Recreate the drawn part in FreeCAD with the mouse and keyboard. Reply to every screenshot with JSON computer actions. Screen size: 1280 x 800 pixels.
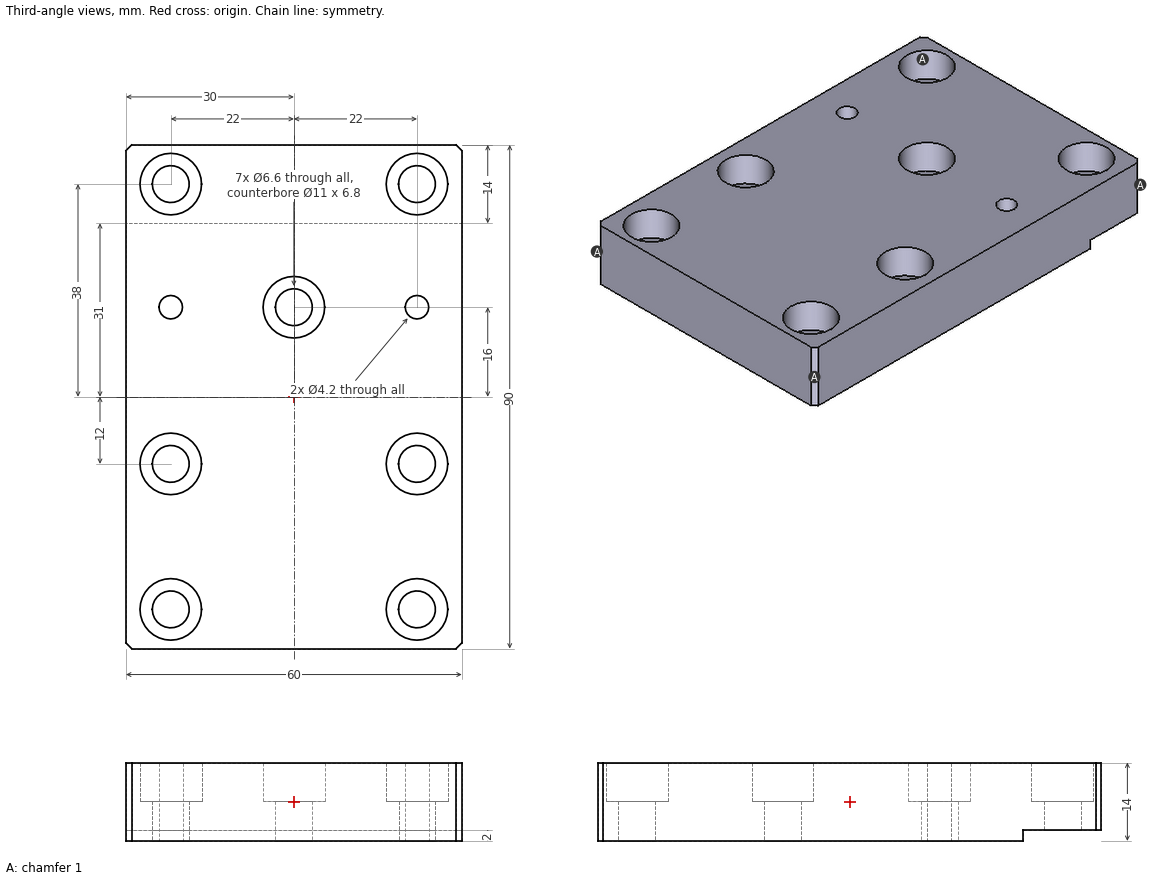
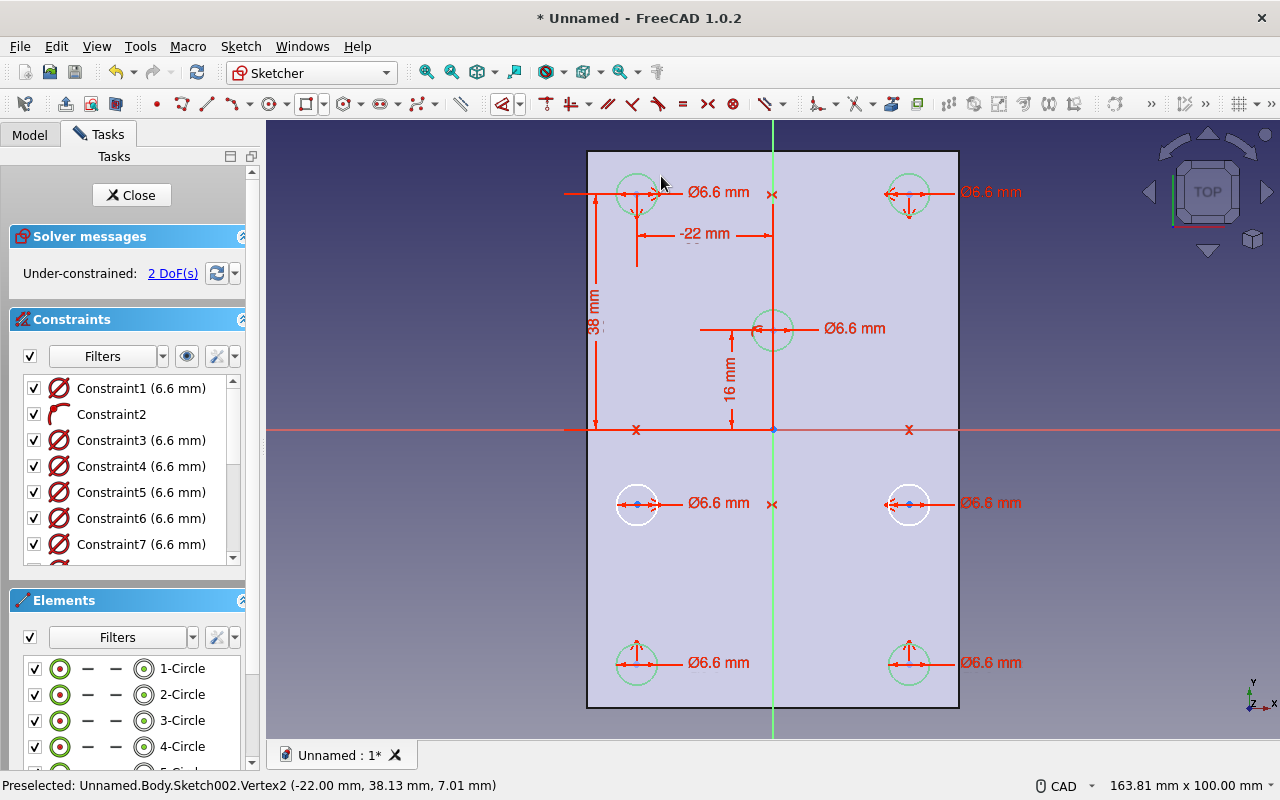
{"action": "left_click", "coordinate": [637, 505]}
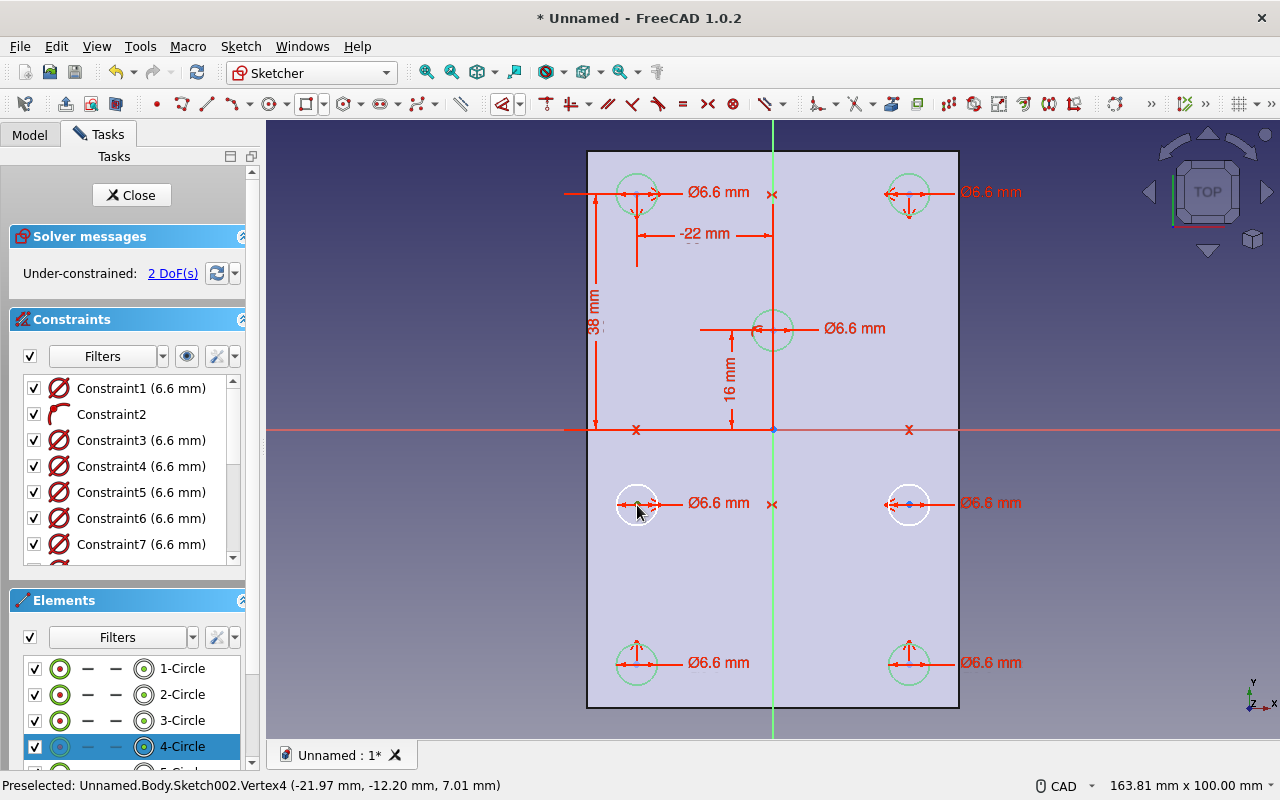
{"action": "left_click", "coordinate": [520, 104]}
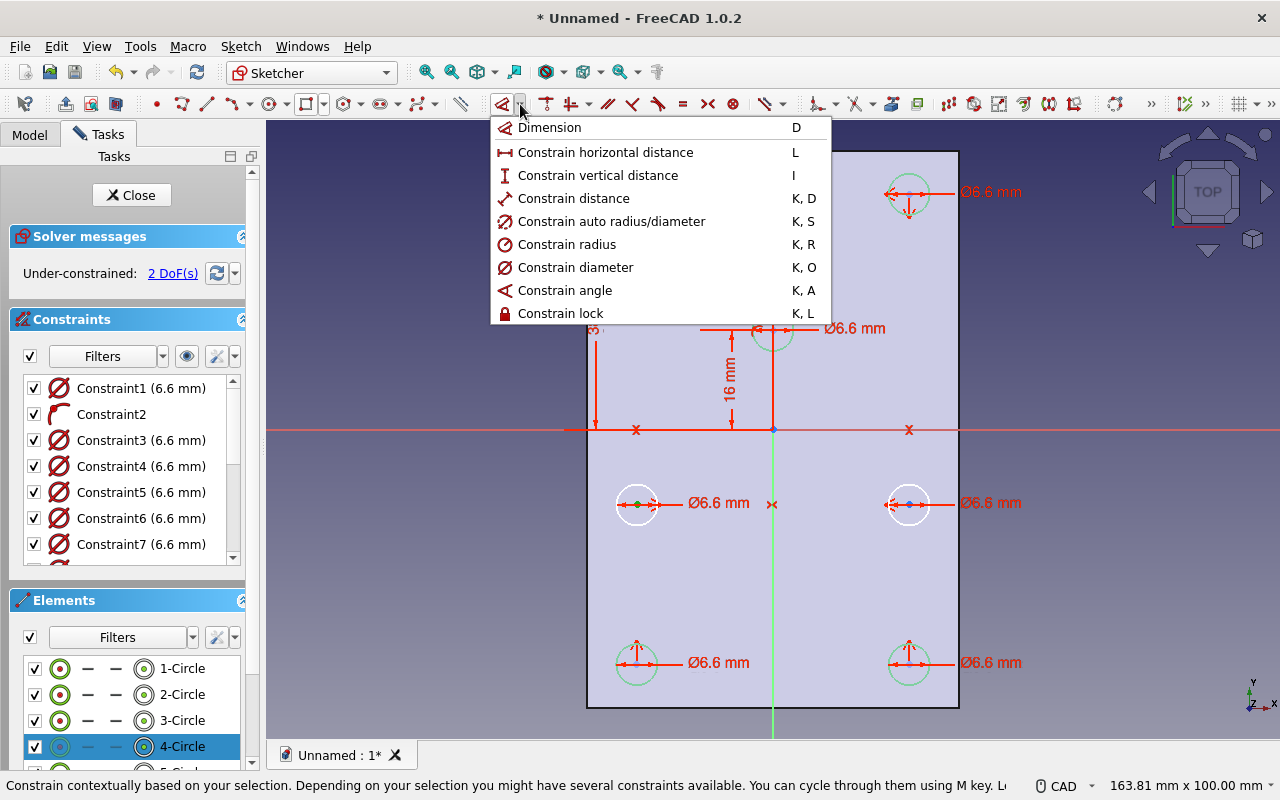
{"action": "left_click", "coordinate": [661, 152]}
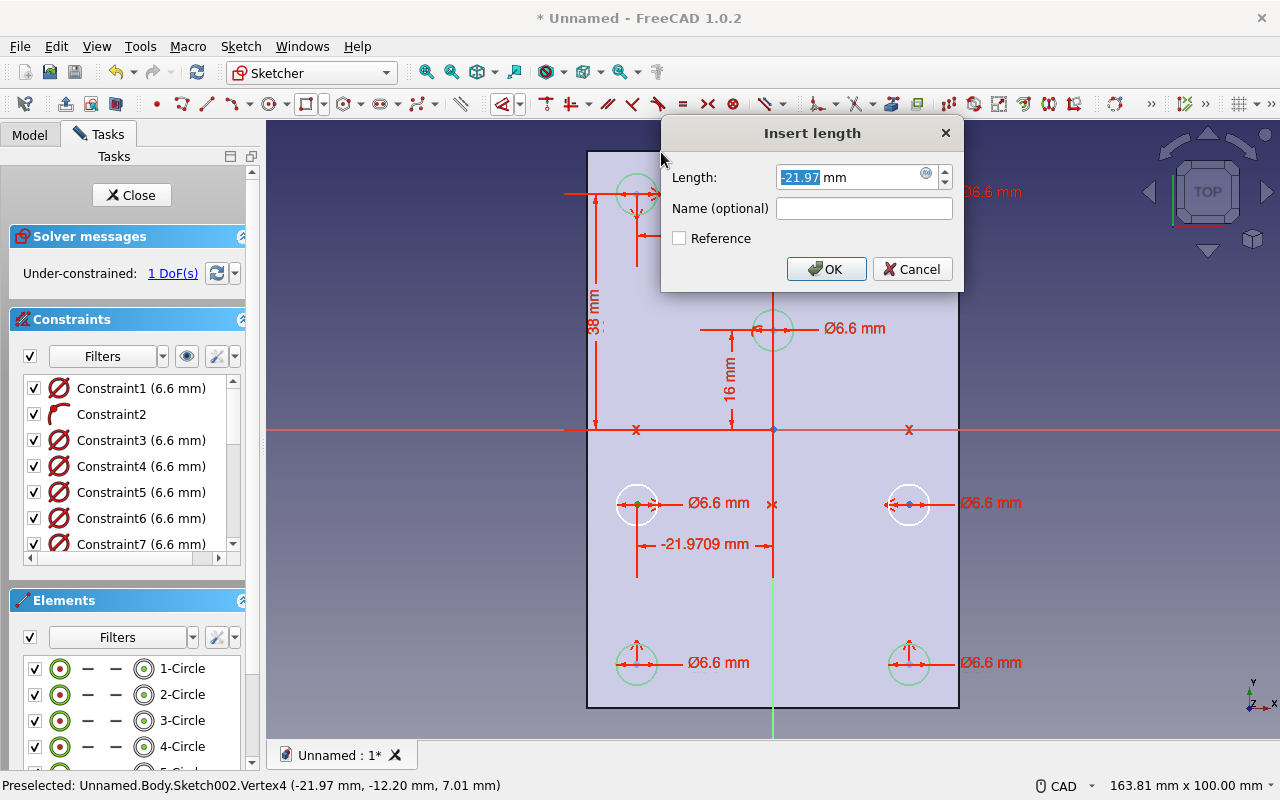
{"action": "type", "text": "-22"}
{"action": "key", "text": "Return"}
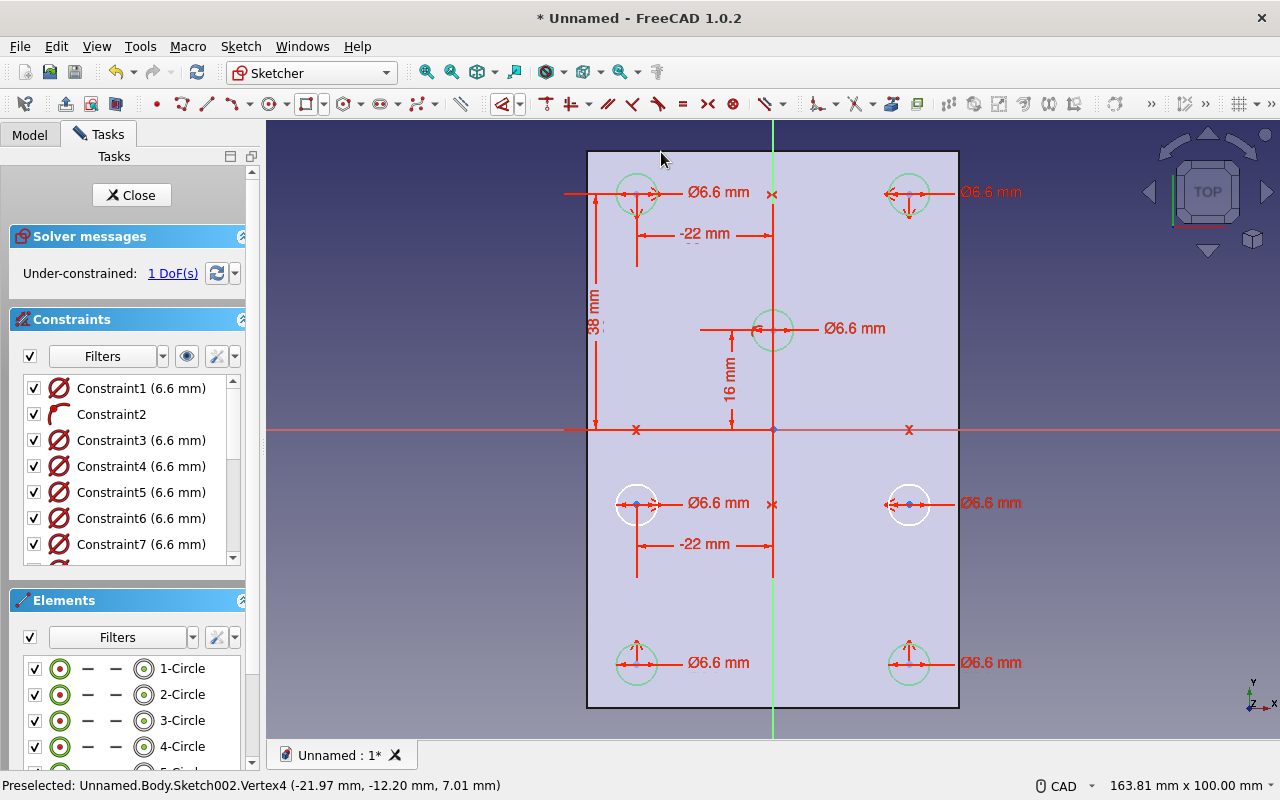
{"action": "left_click", "coordinate": [637, 505]}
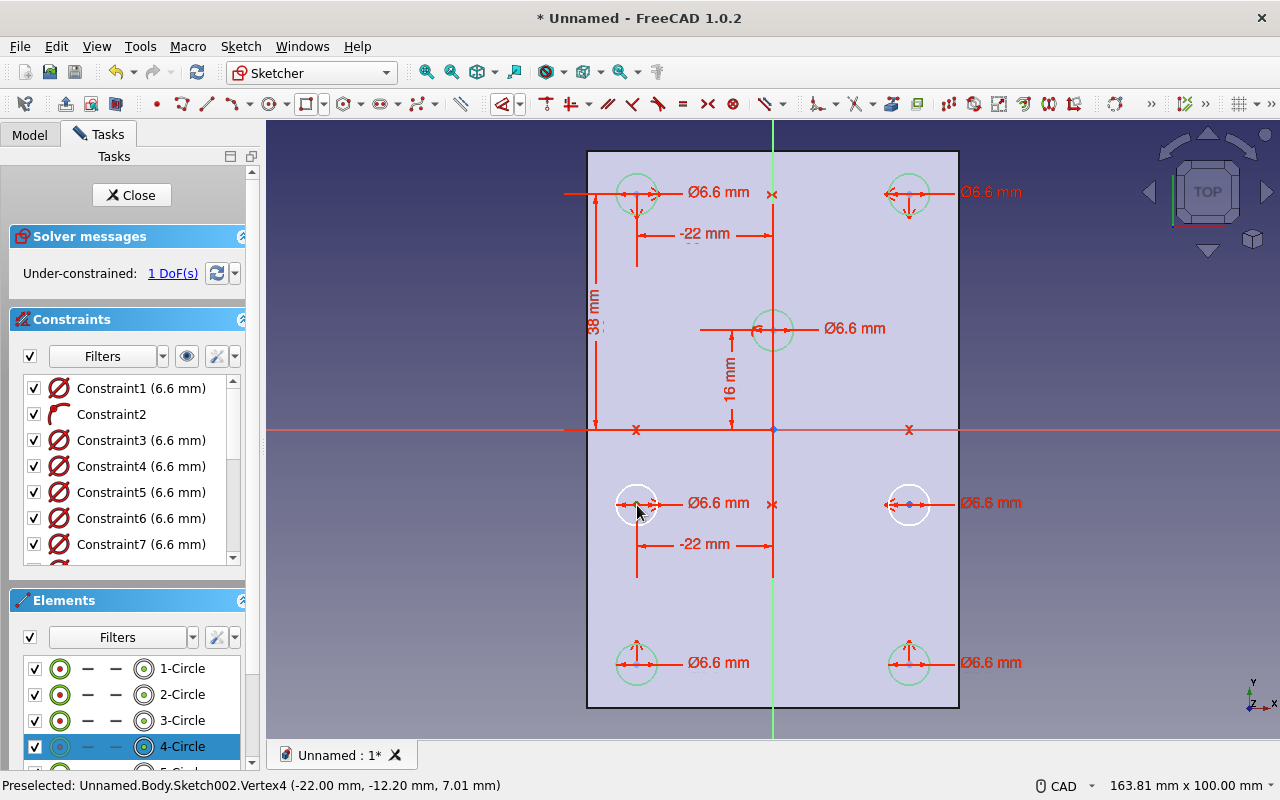
{"action": "left_click", "coordinate": [520, 104]}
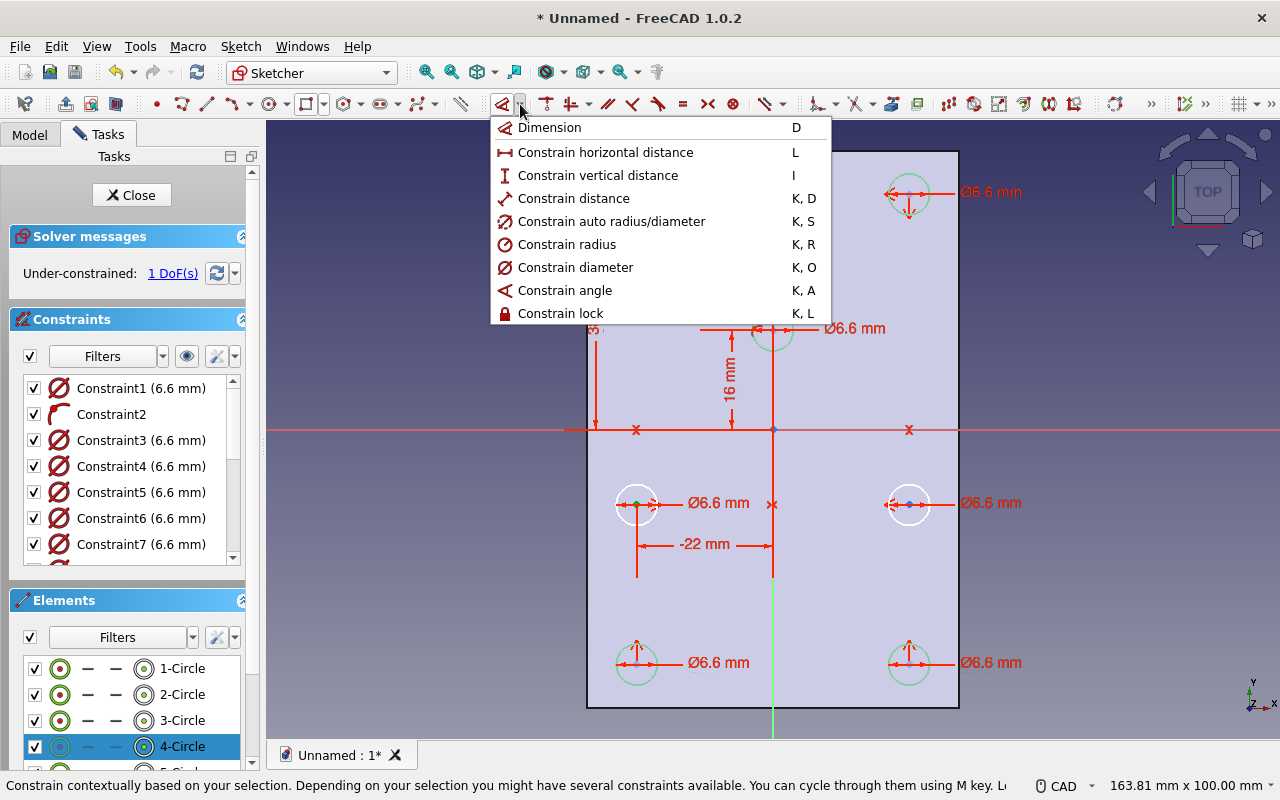
{"action": "left_click", "coordinate": [661, 176]}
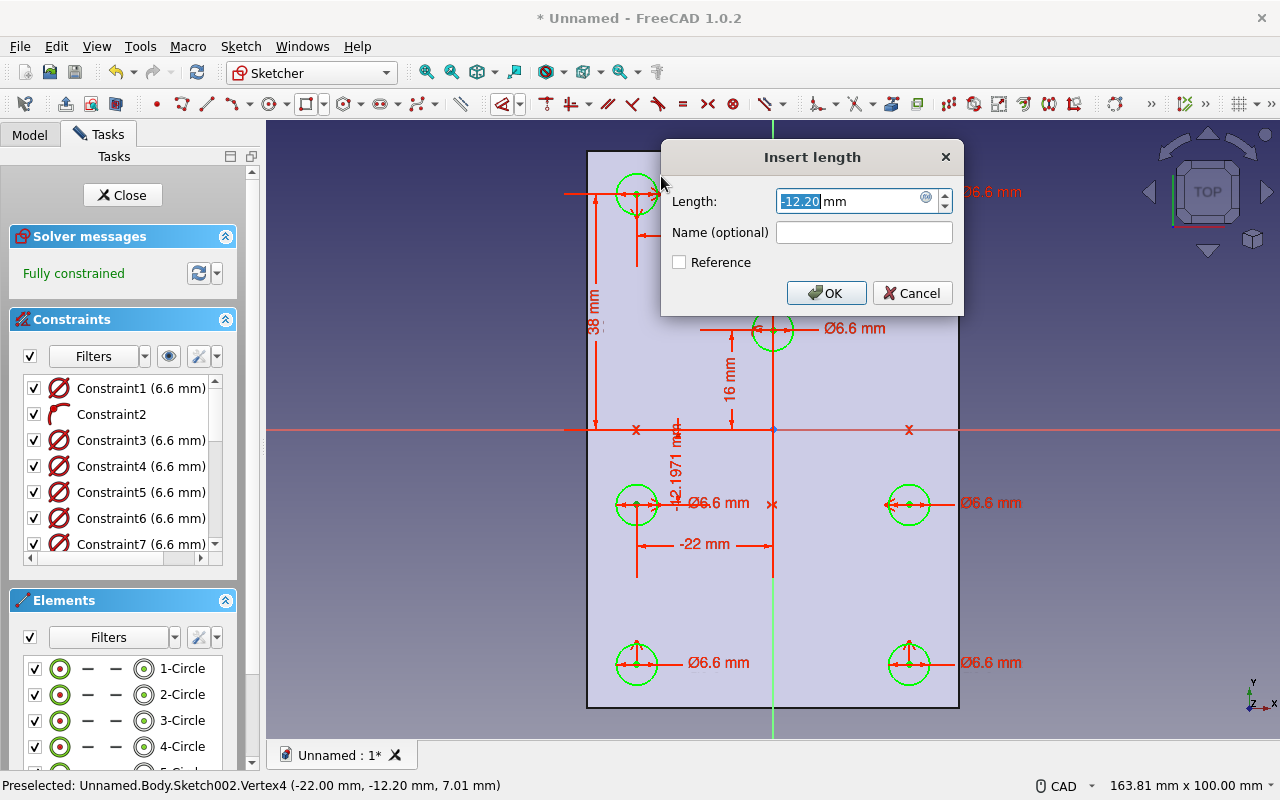
{"action": "type", "text": "-12"}
{"action": "key", "text": "Return"}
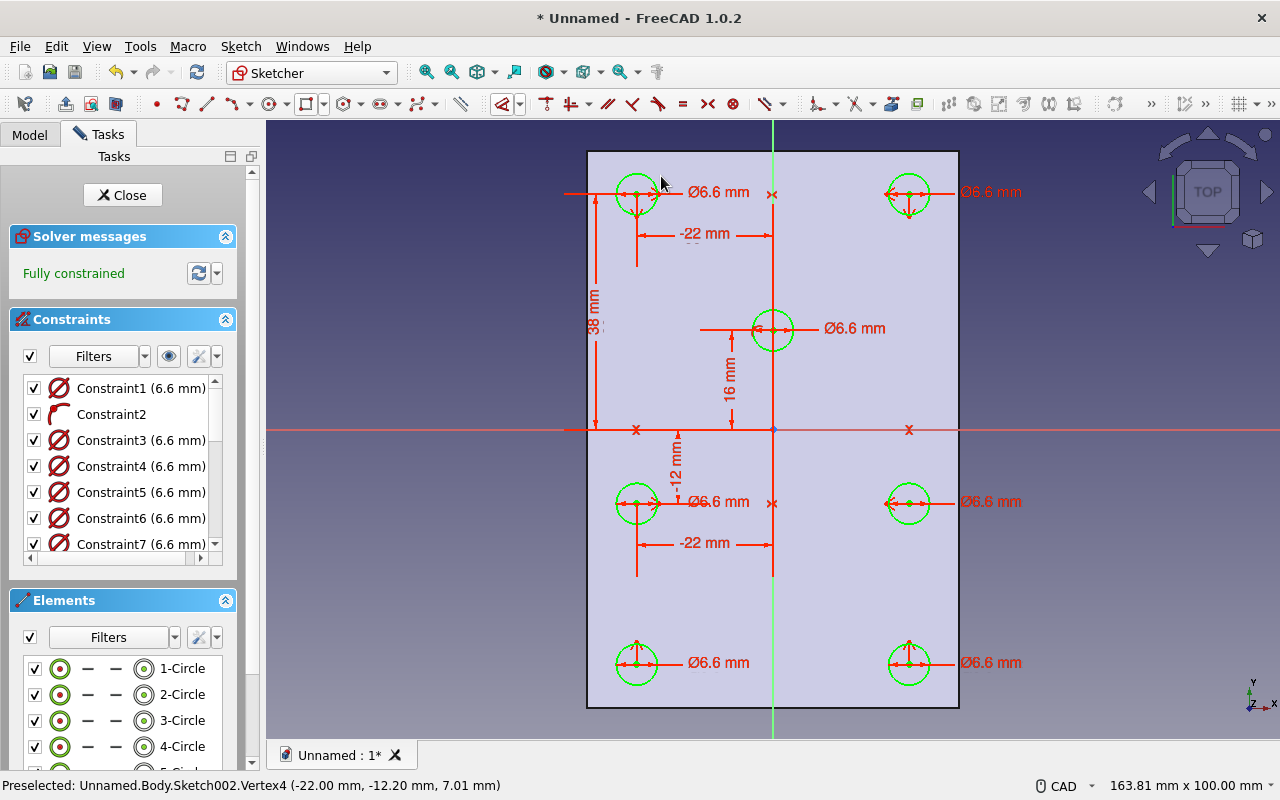
{"action": "left_click", "coordinate": [123, 195]}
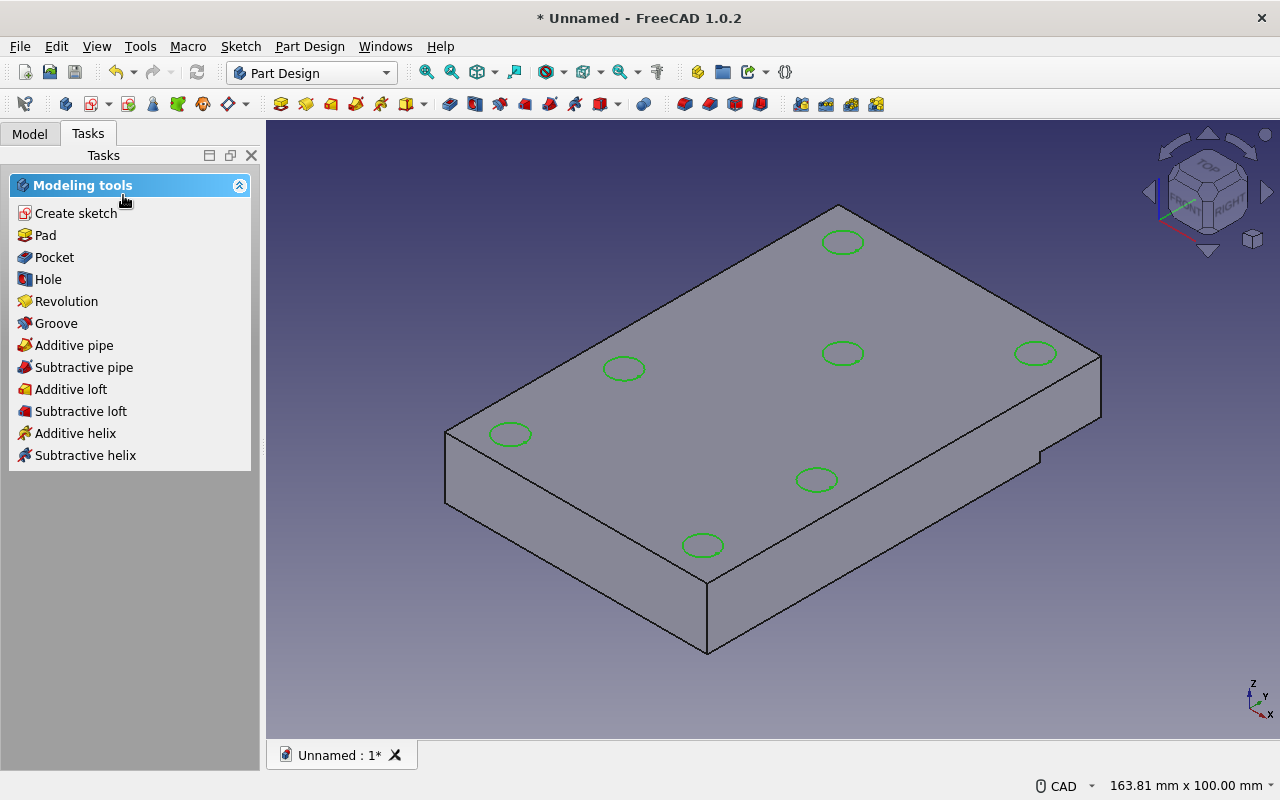
{"action": "left_click", "coordinate": [475, 104]}